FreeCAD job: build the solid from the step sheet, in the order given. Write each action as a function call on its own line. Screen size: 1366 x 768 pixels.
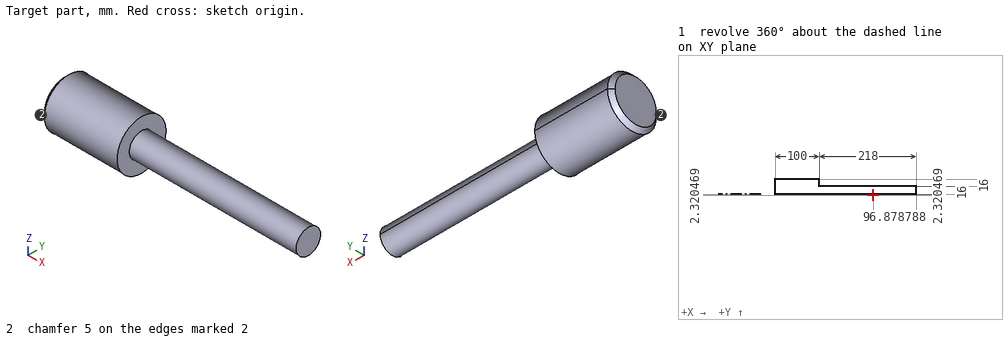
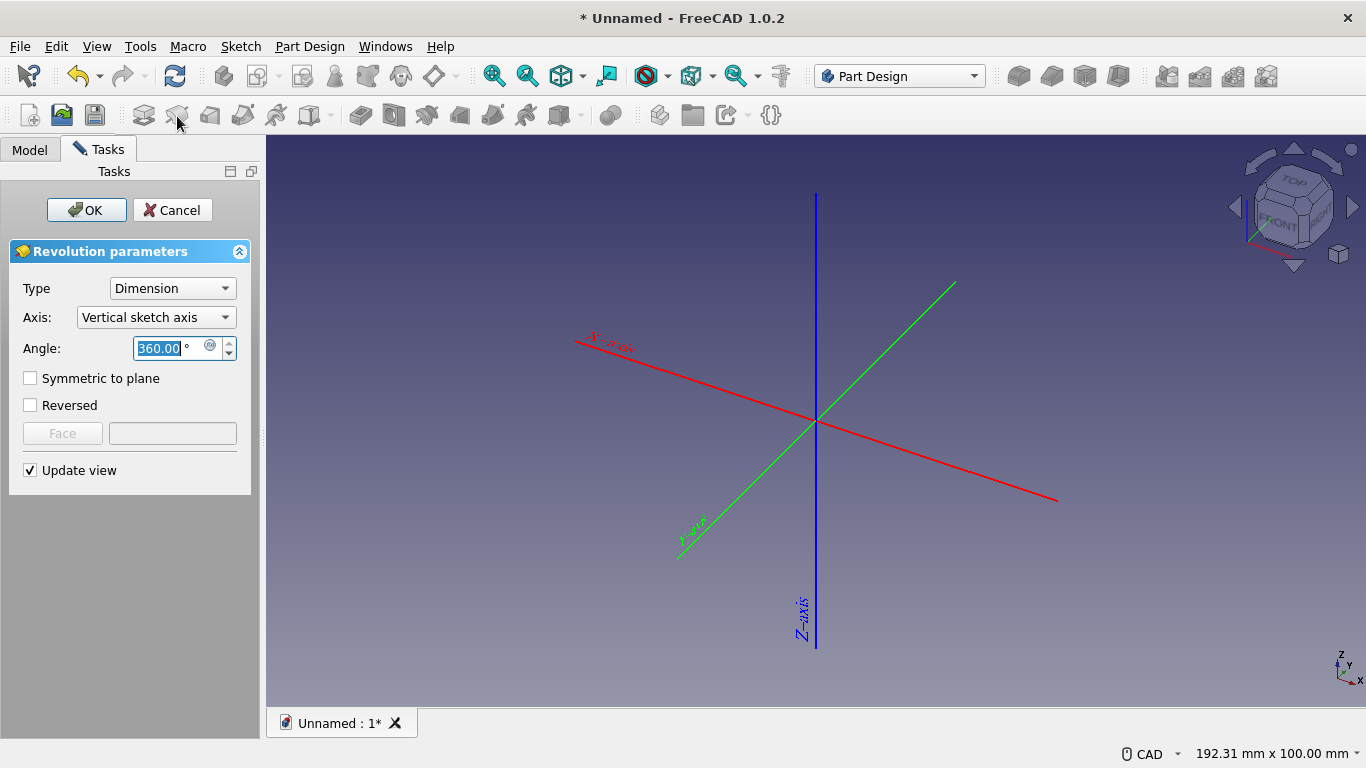
click(157, 318)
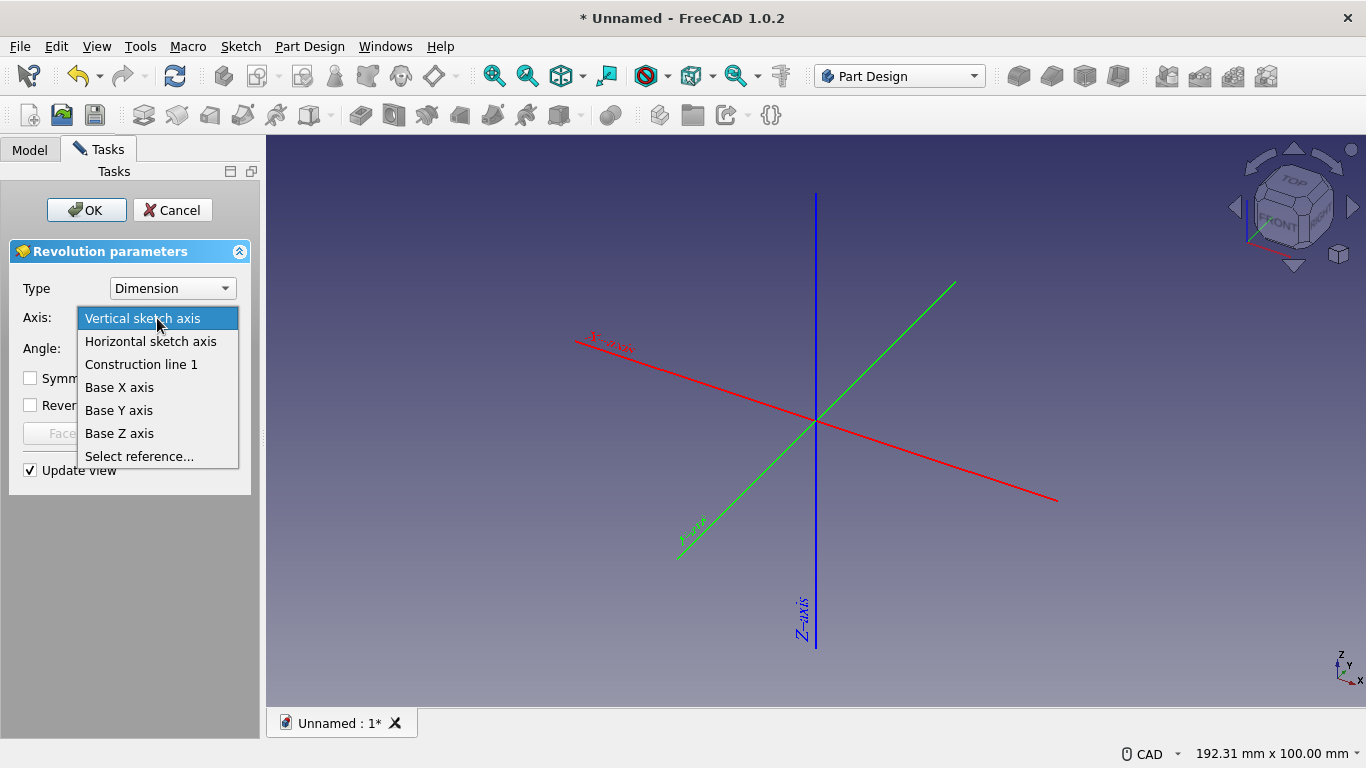
click(156, 364)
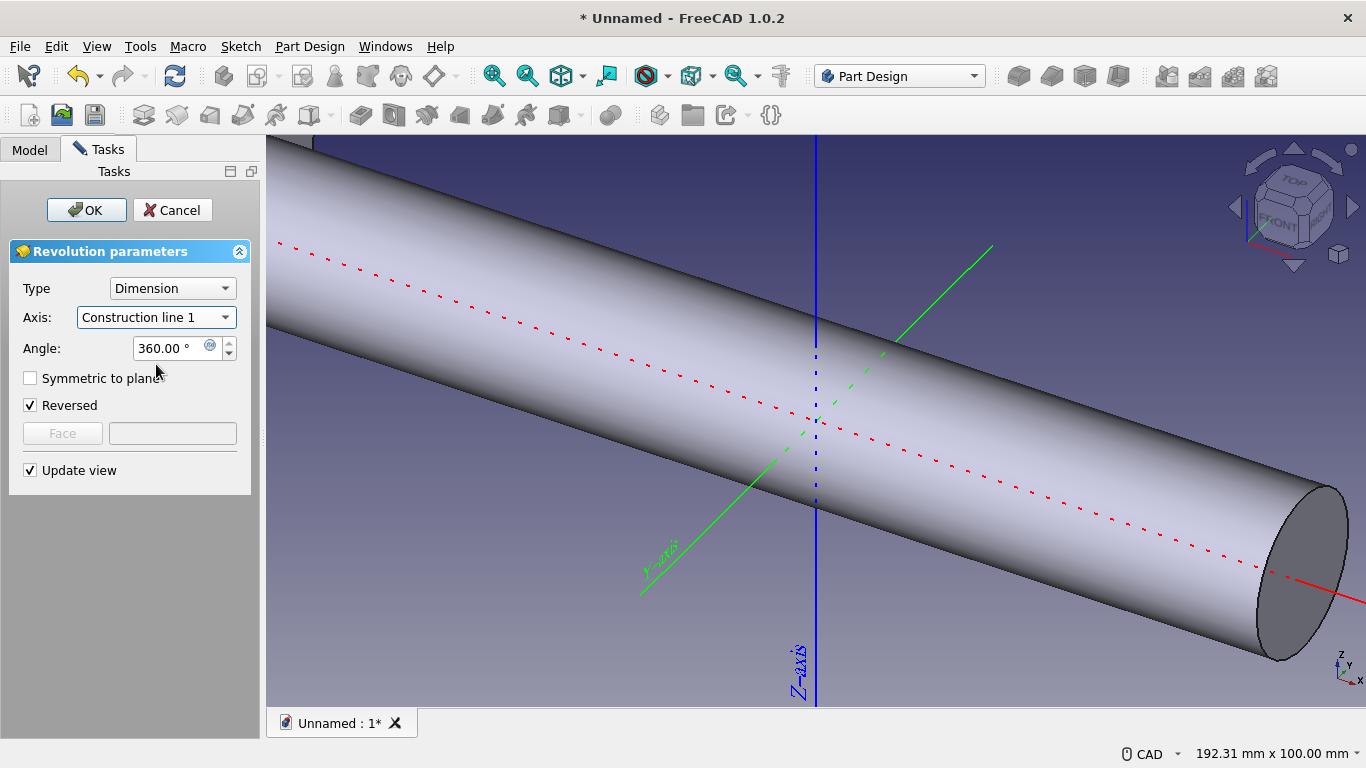
click(87, 210)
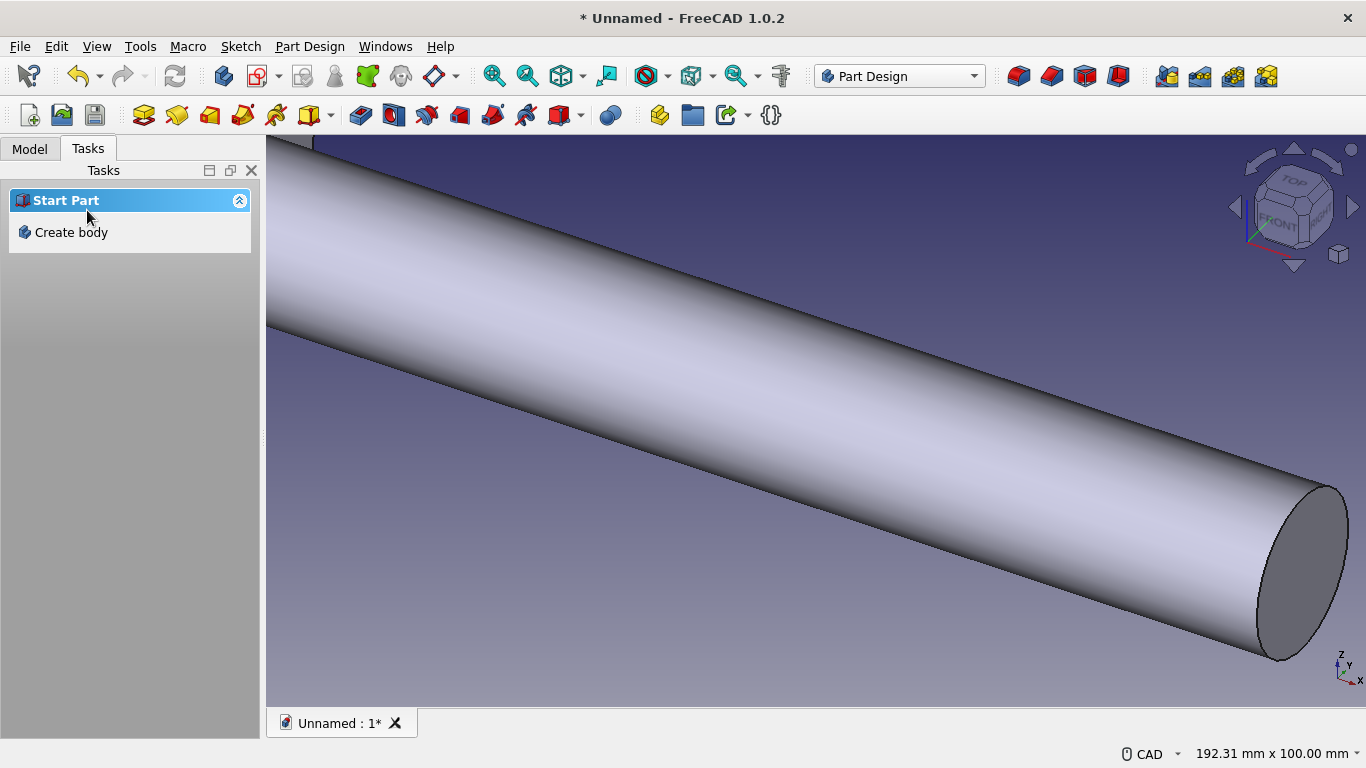
key(v)
key(f)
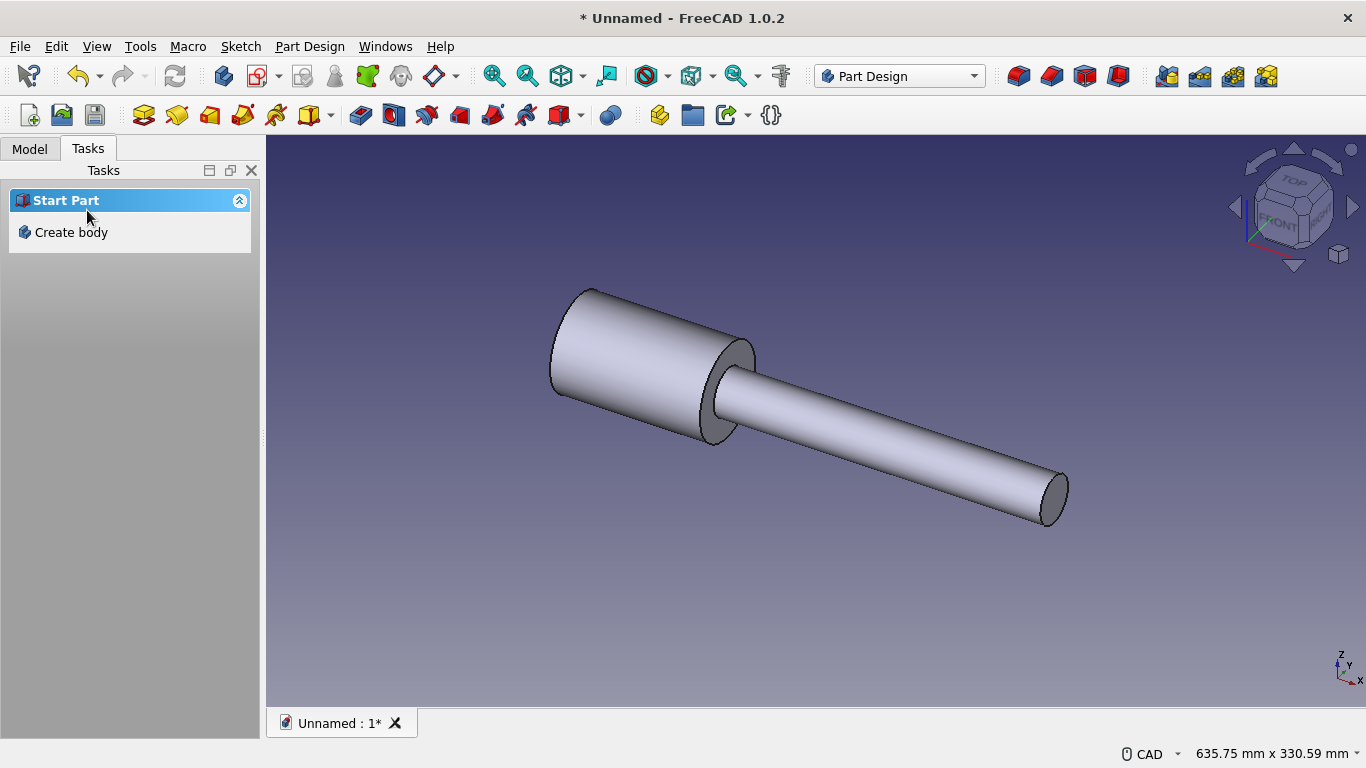
key(0)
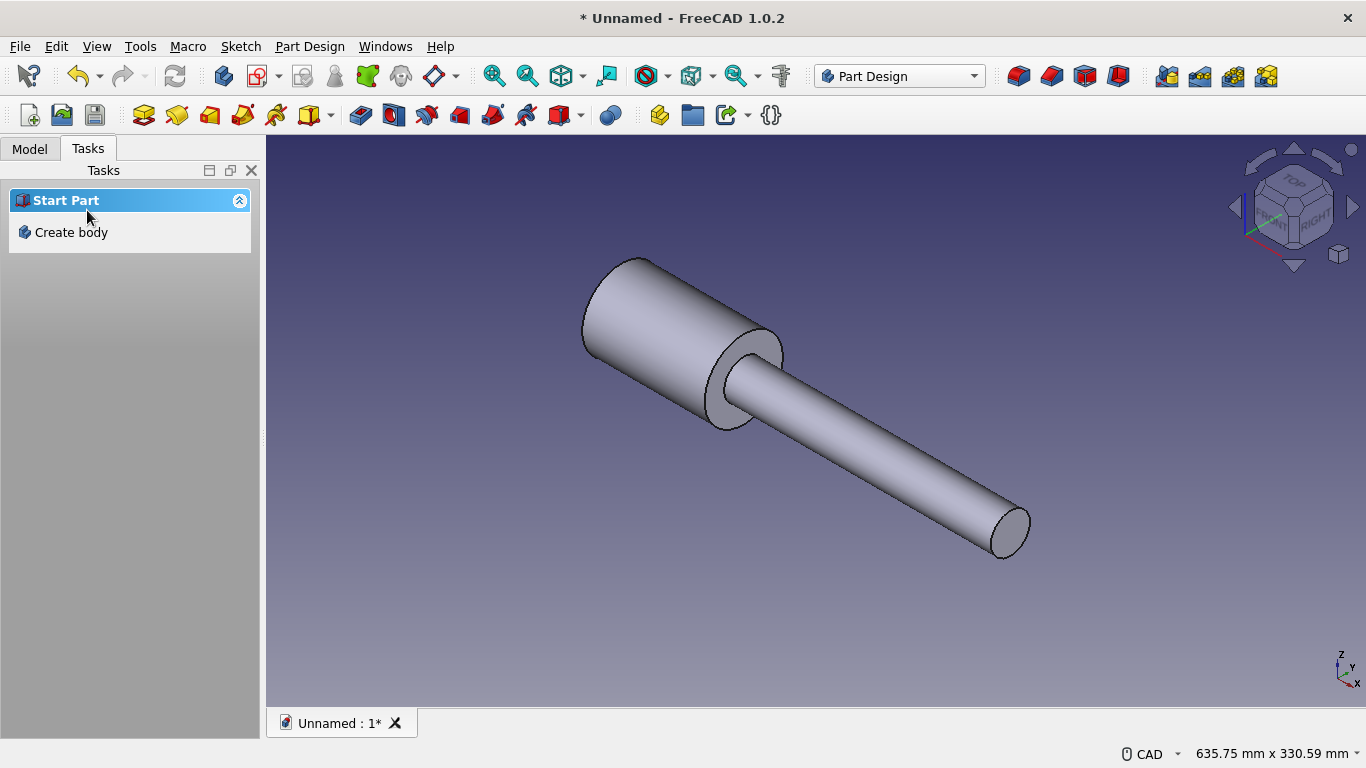
key(2)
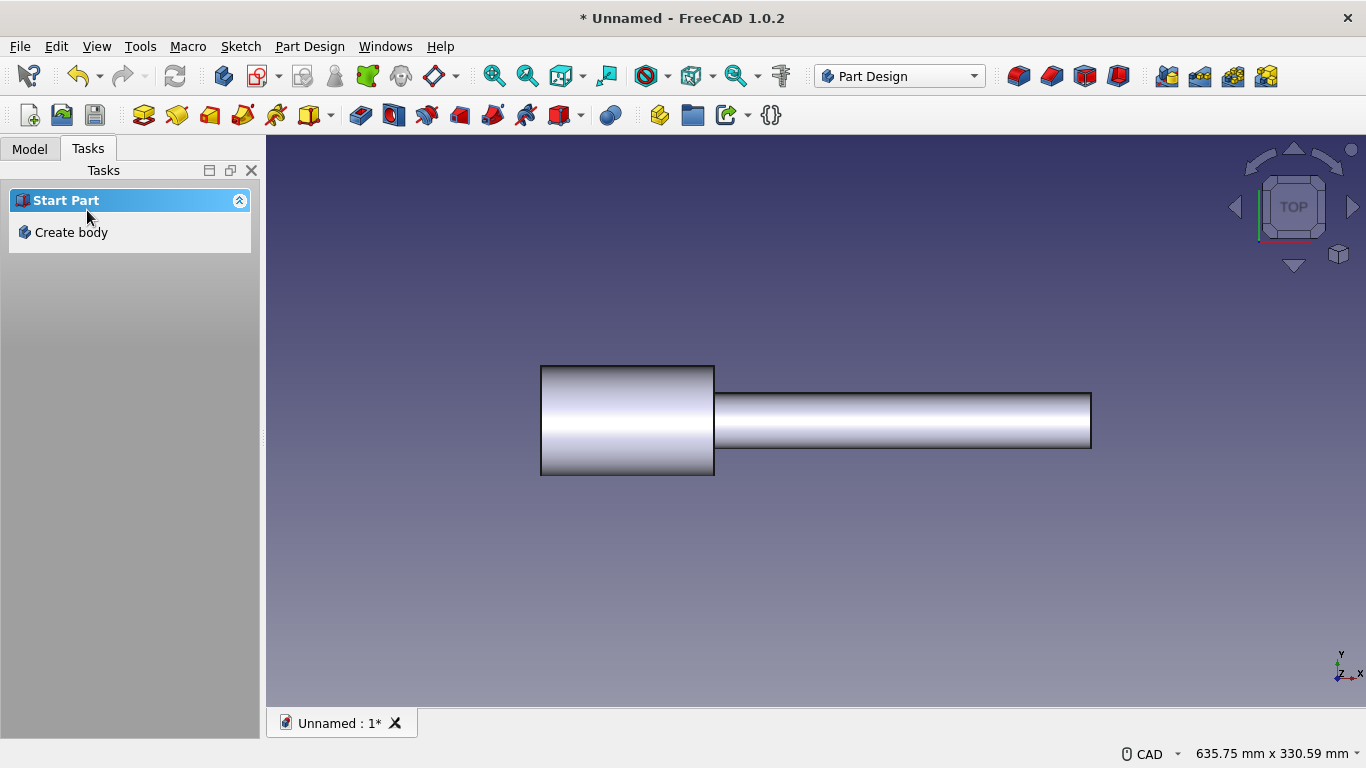
click(541, 475)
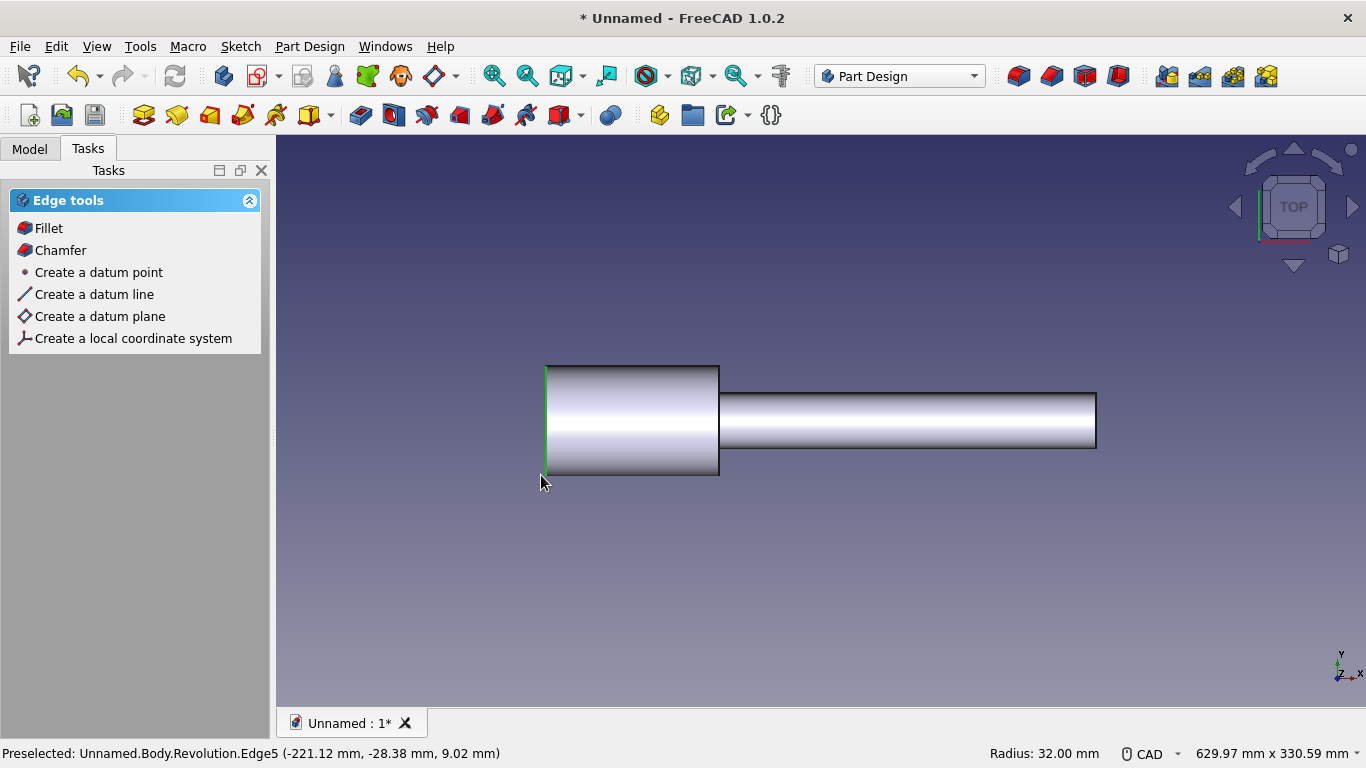
click(1052, 76)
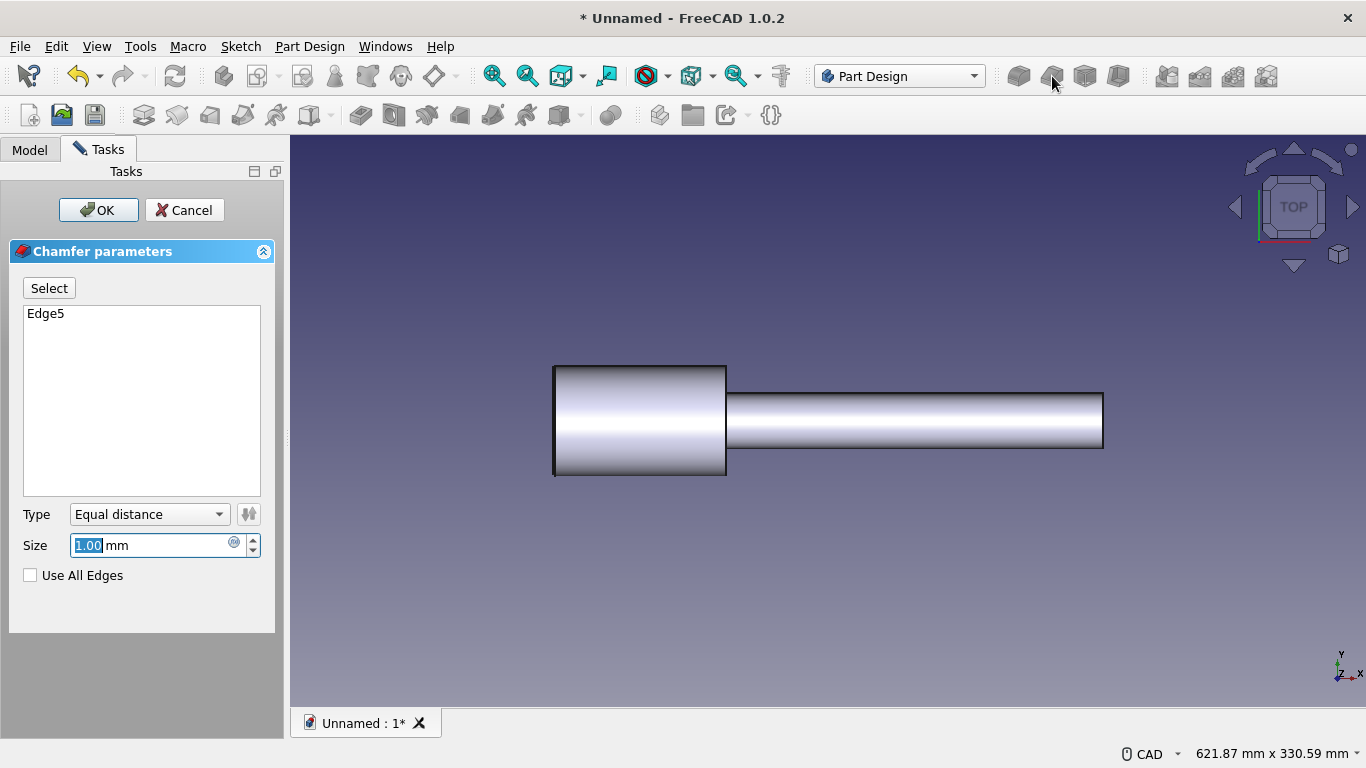
text(5)
key(Tab)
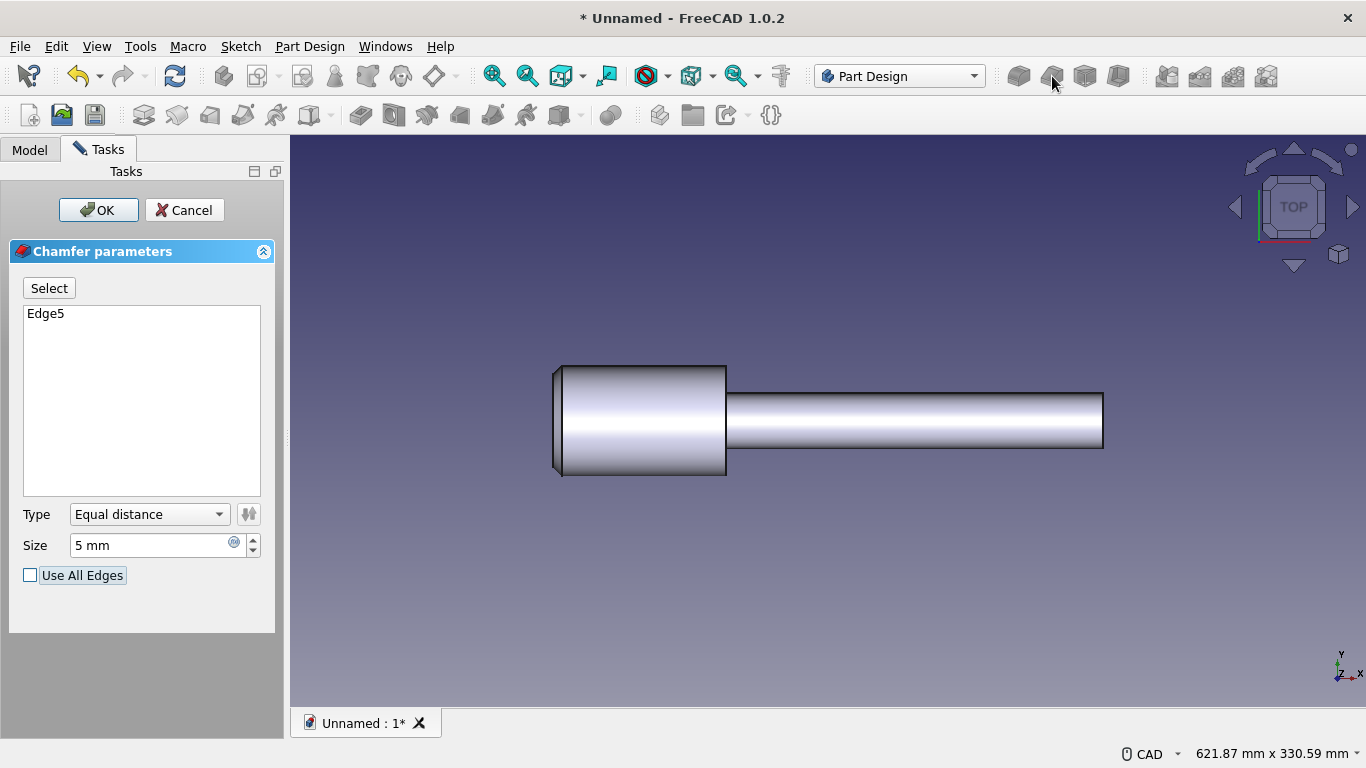
click(99, 210)